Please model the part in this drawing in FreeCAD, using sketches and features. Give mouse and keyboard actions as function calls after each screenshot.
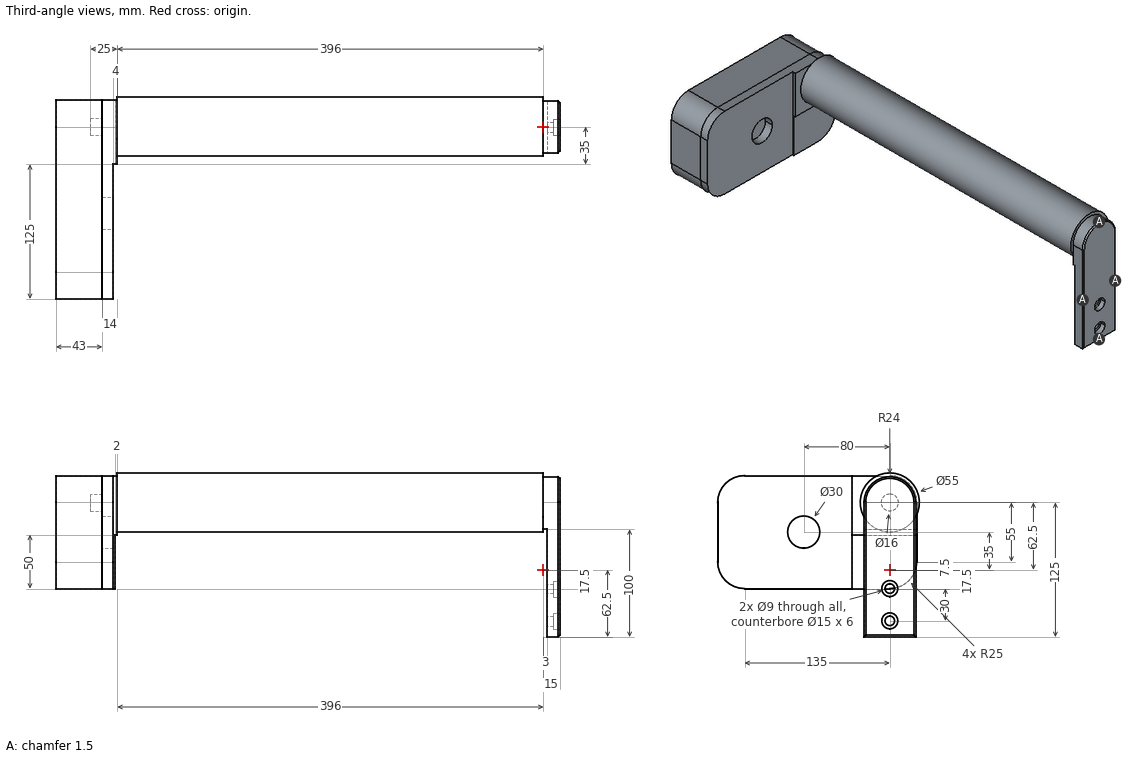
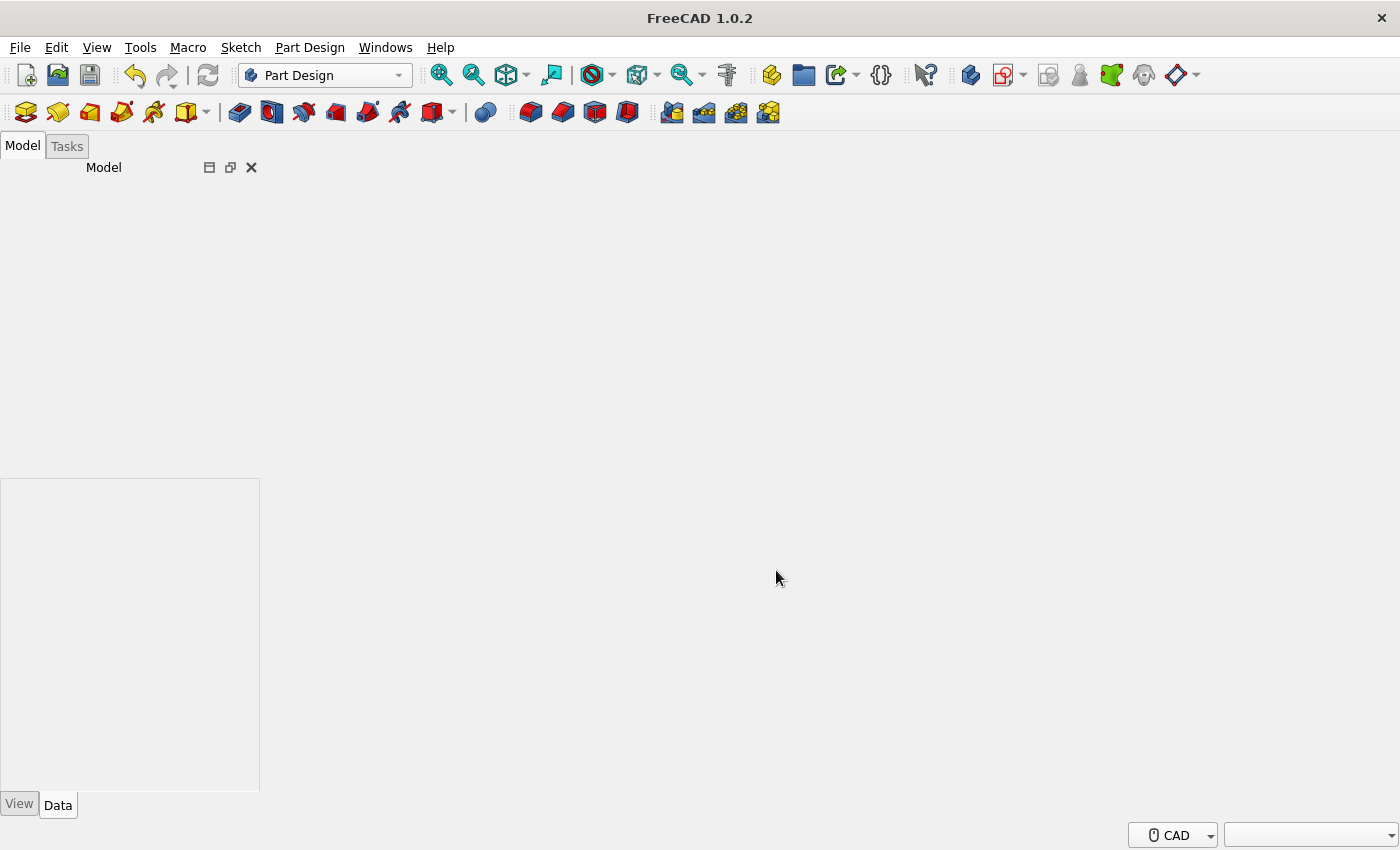
click(26, 76)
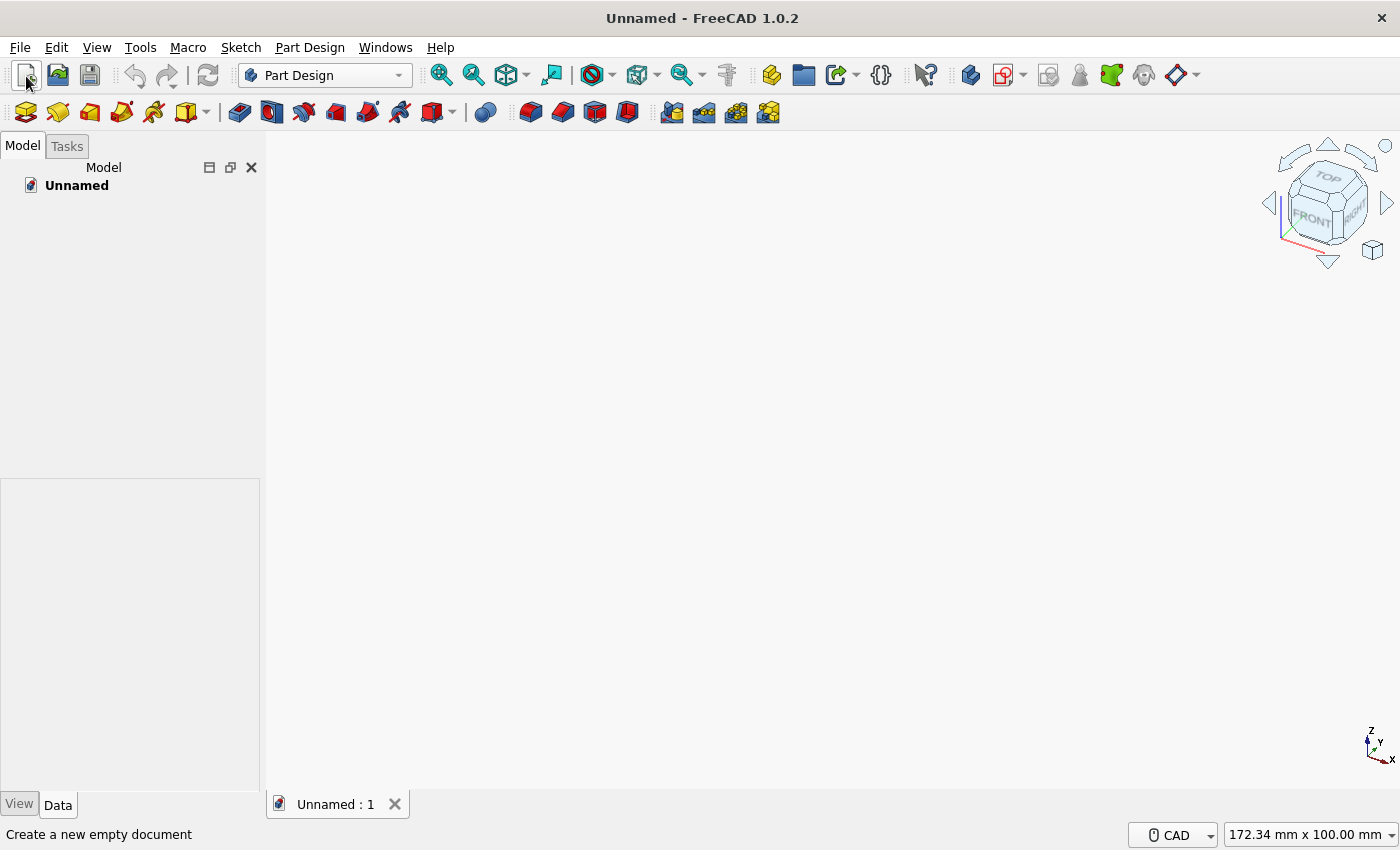
click(1004, 76)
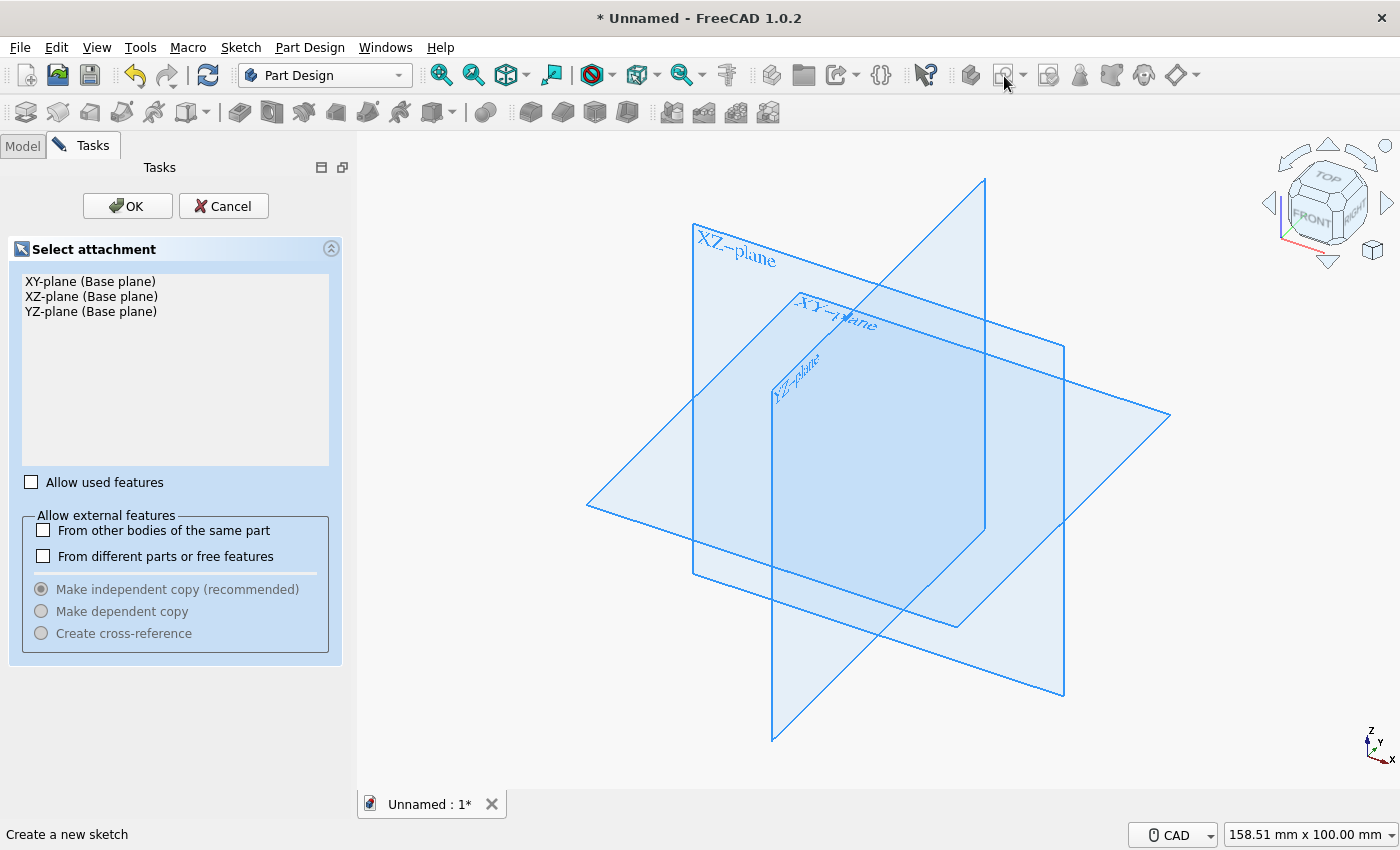
click(82, 312)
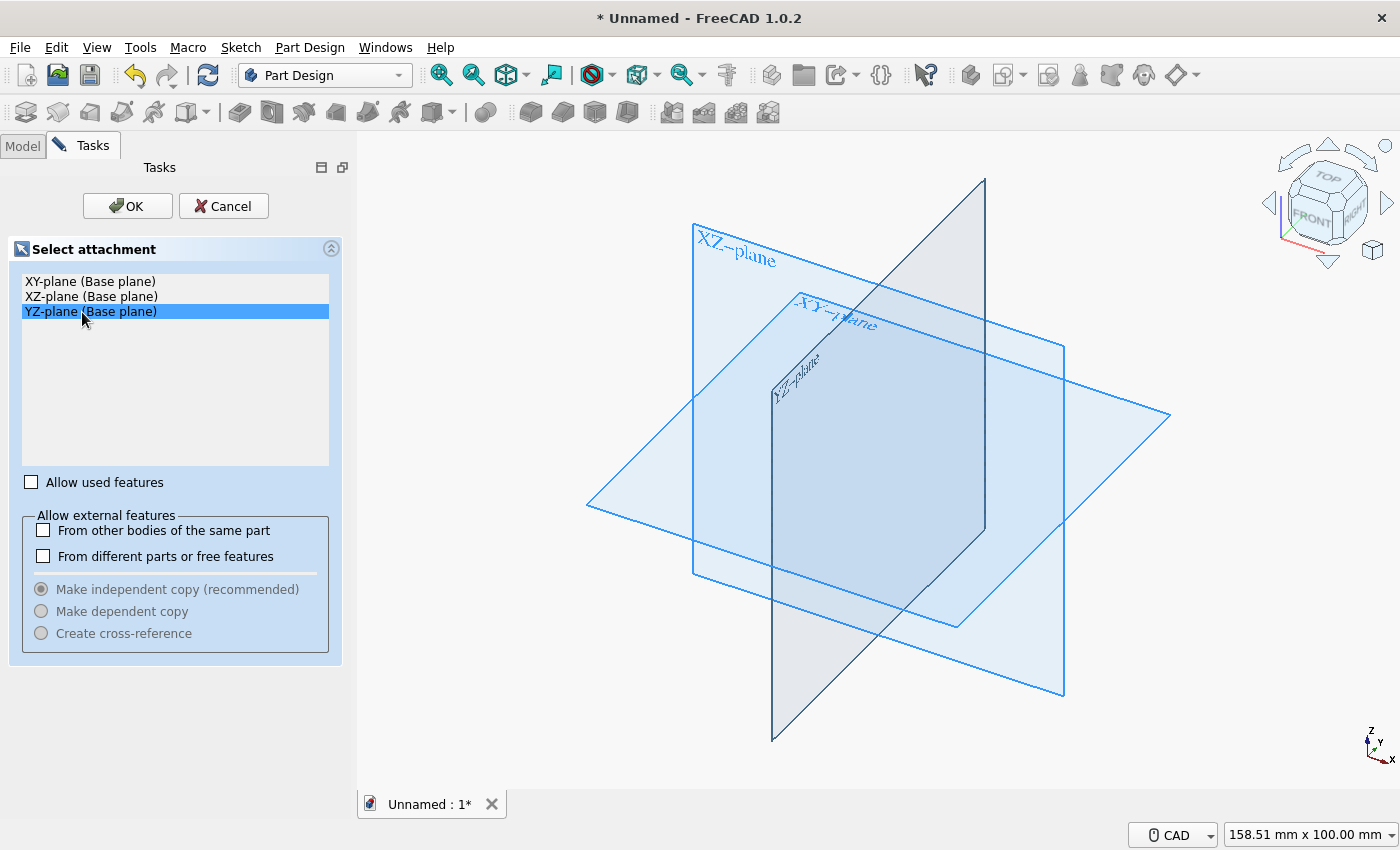
click(128, 206)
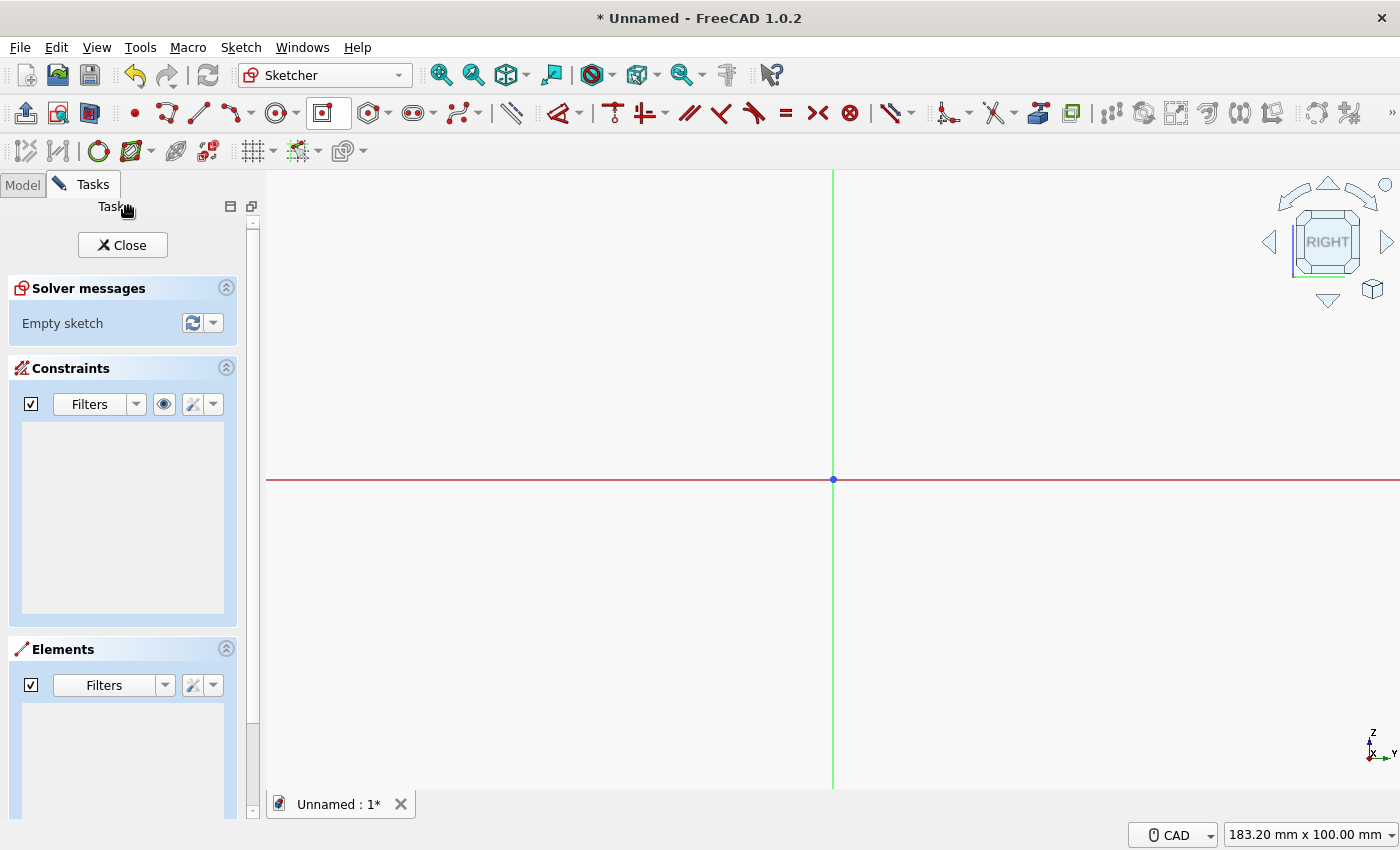
scroll(709, 540, down, 4)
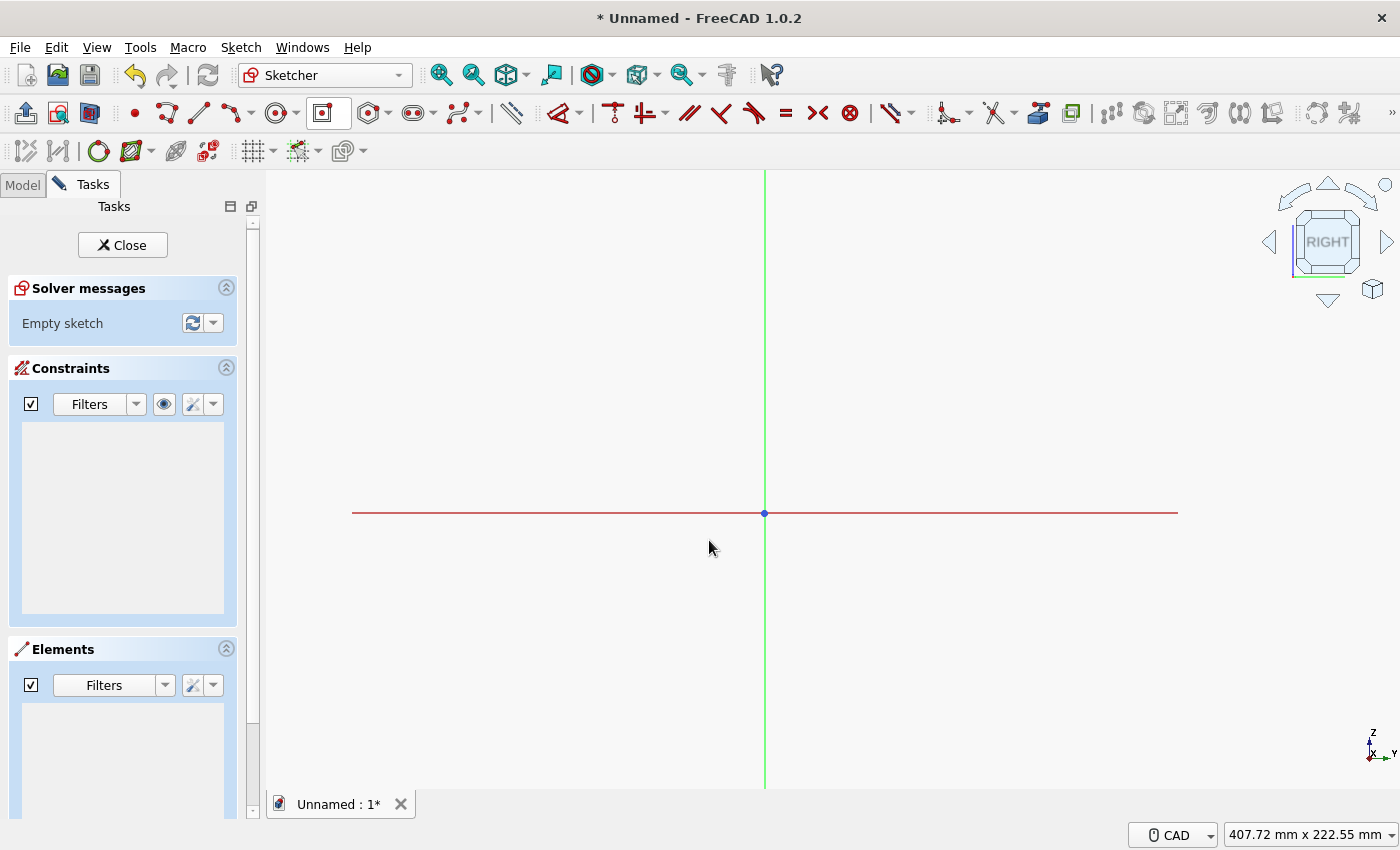
key(g)
key(m)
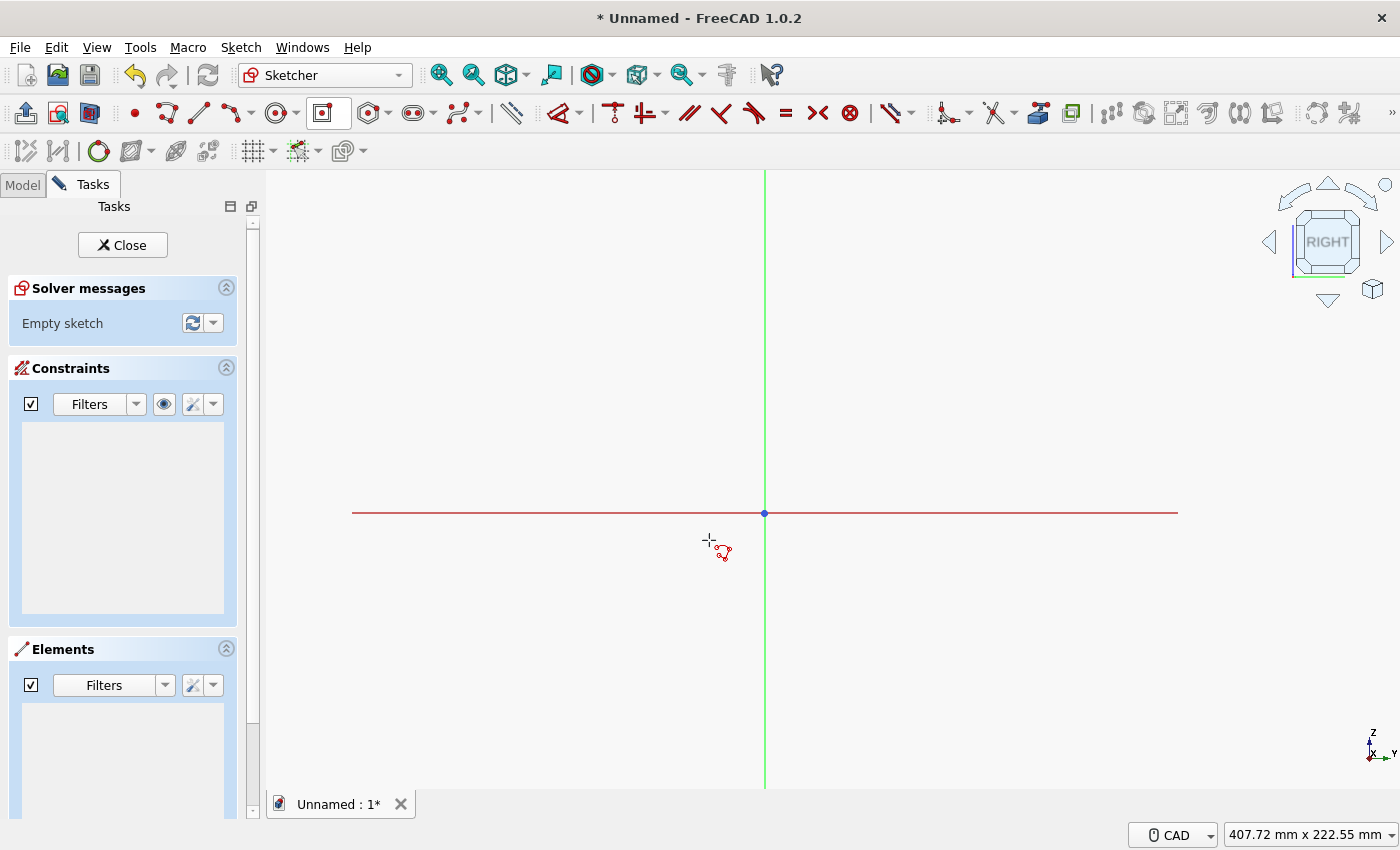
click(698, 339)
click(698, 687)
click(832, 687)
click(832, 339)
right_click(832, 339)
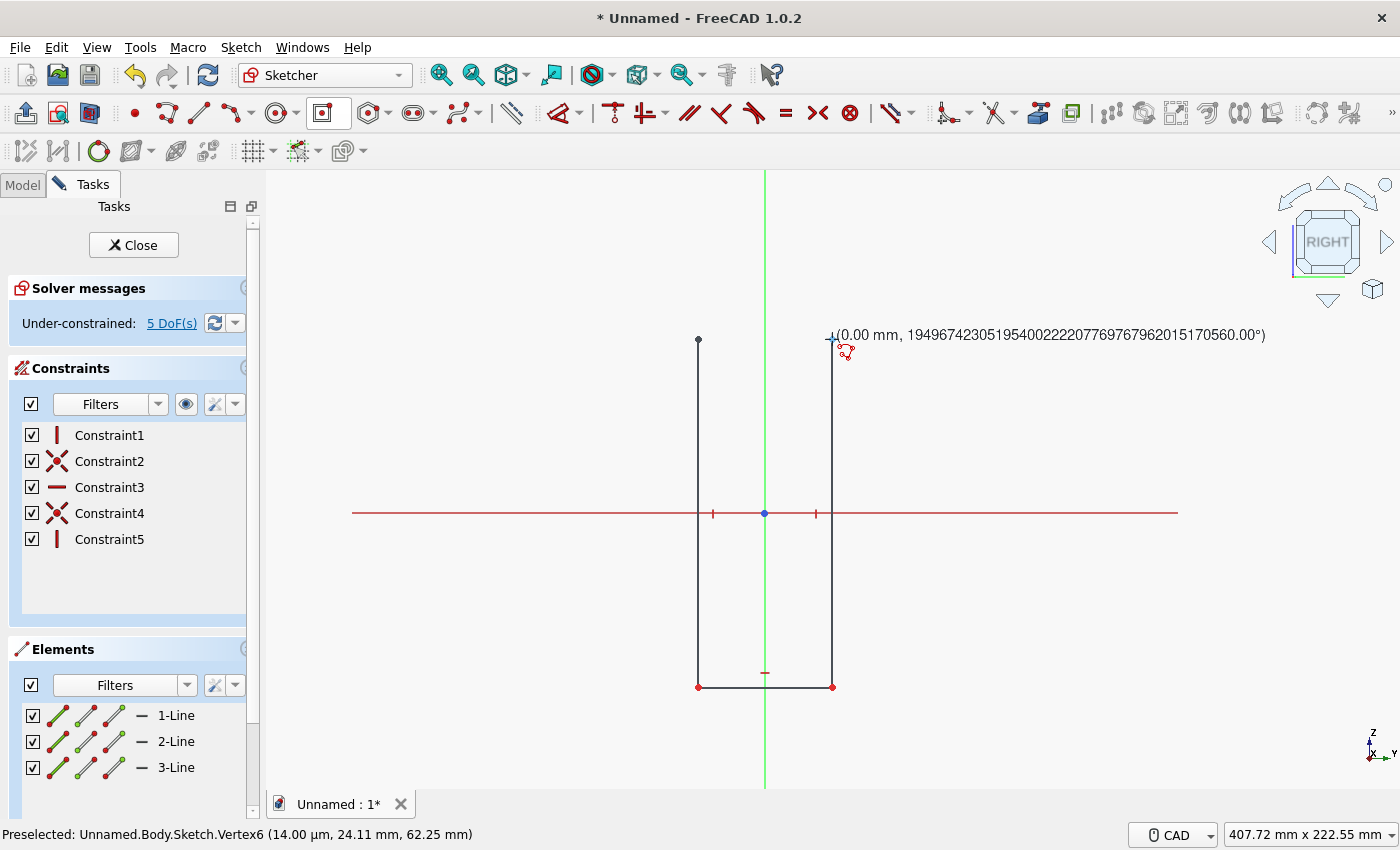
key(g)
key(3)
key(a)